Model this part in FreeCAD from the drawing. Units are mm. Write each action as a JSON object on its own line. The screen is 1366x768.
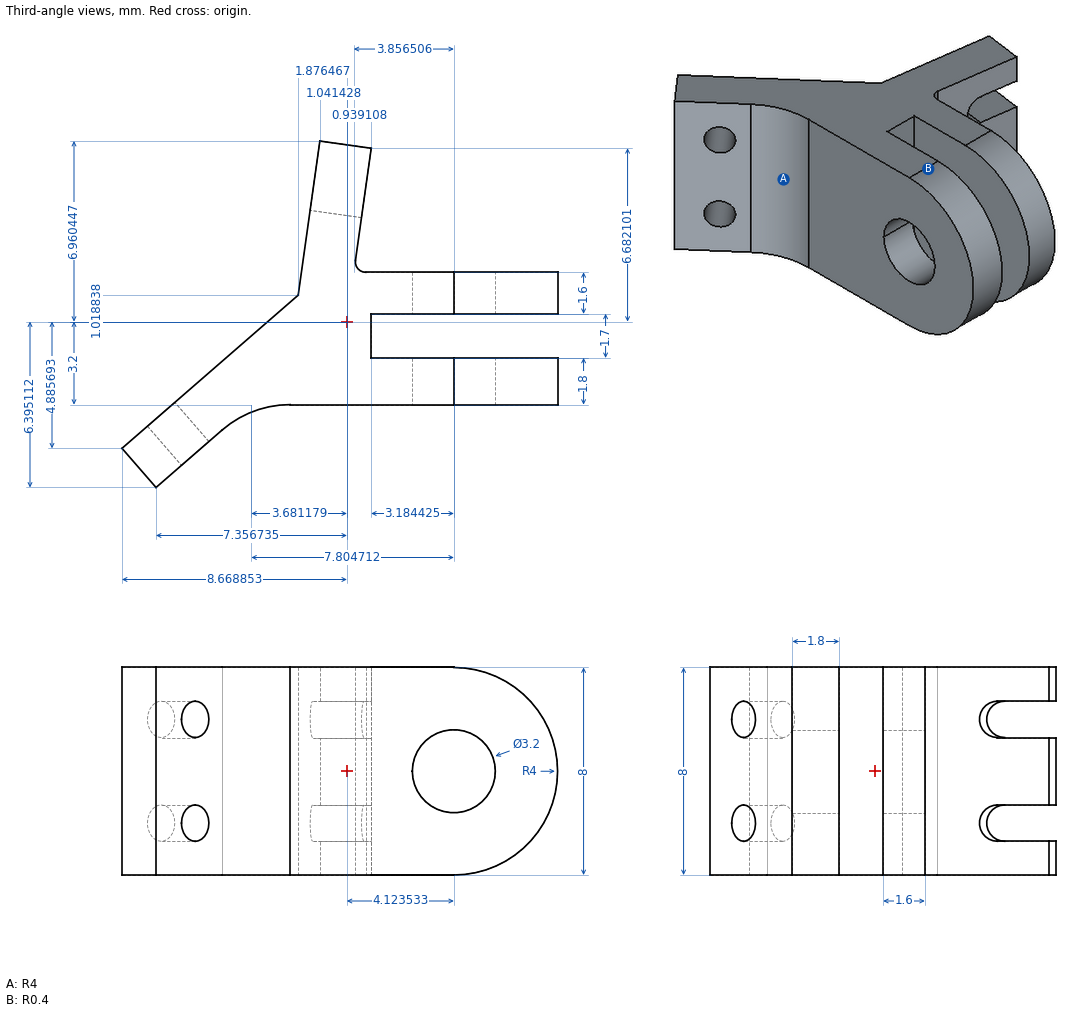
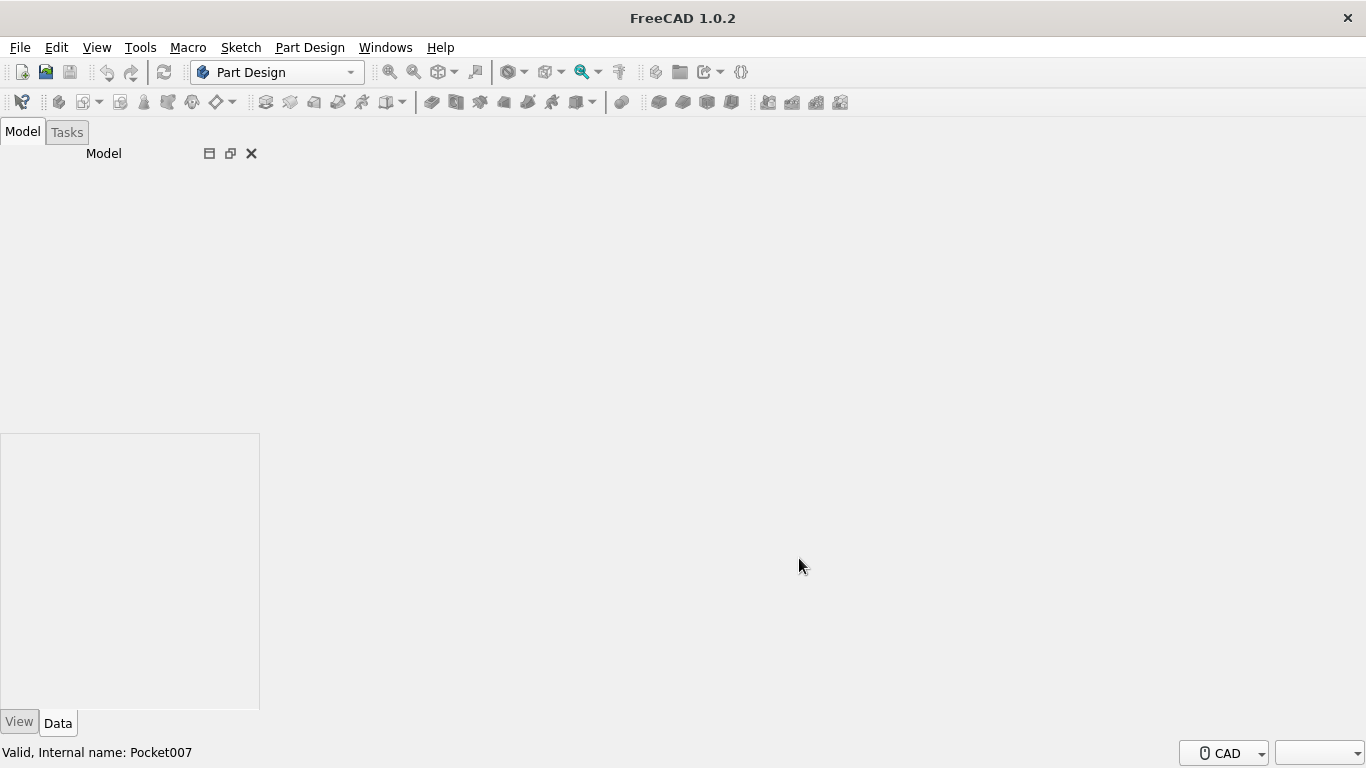
{"action": "left_click", "coordinate": [22, 72]}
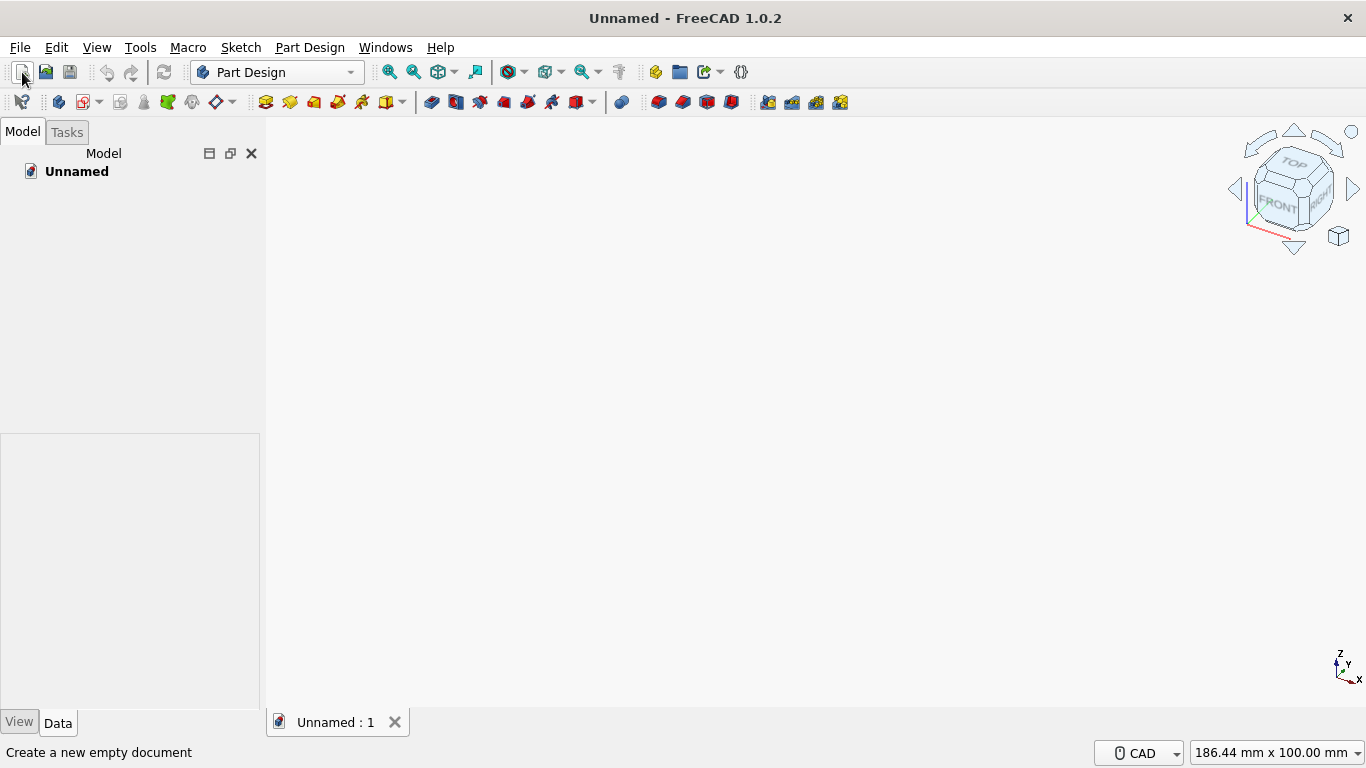
{"action": "left_click", "coordinate": [84, 102]}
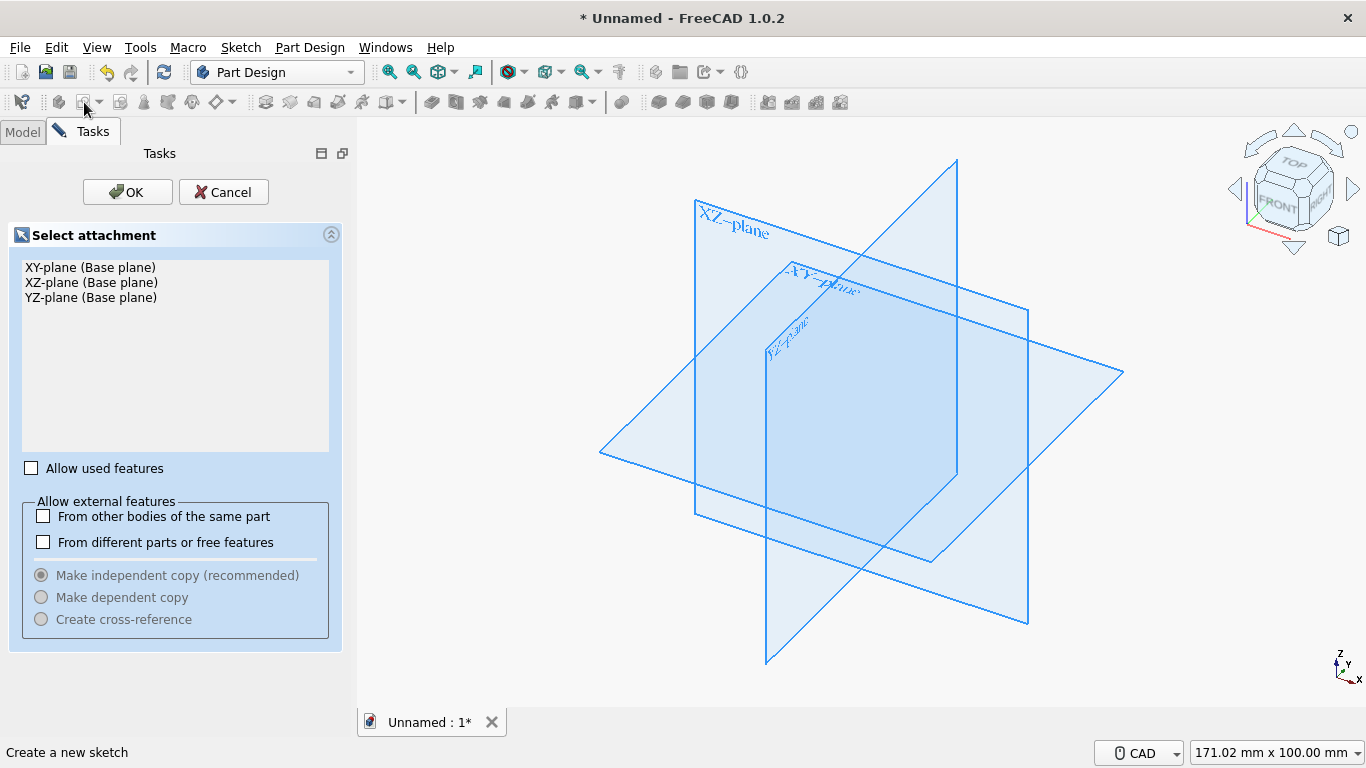
{"action": "left_click", "coordinate": [82, 268]}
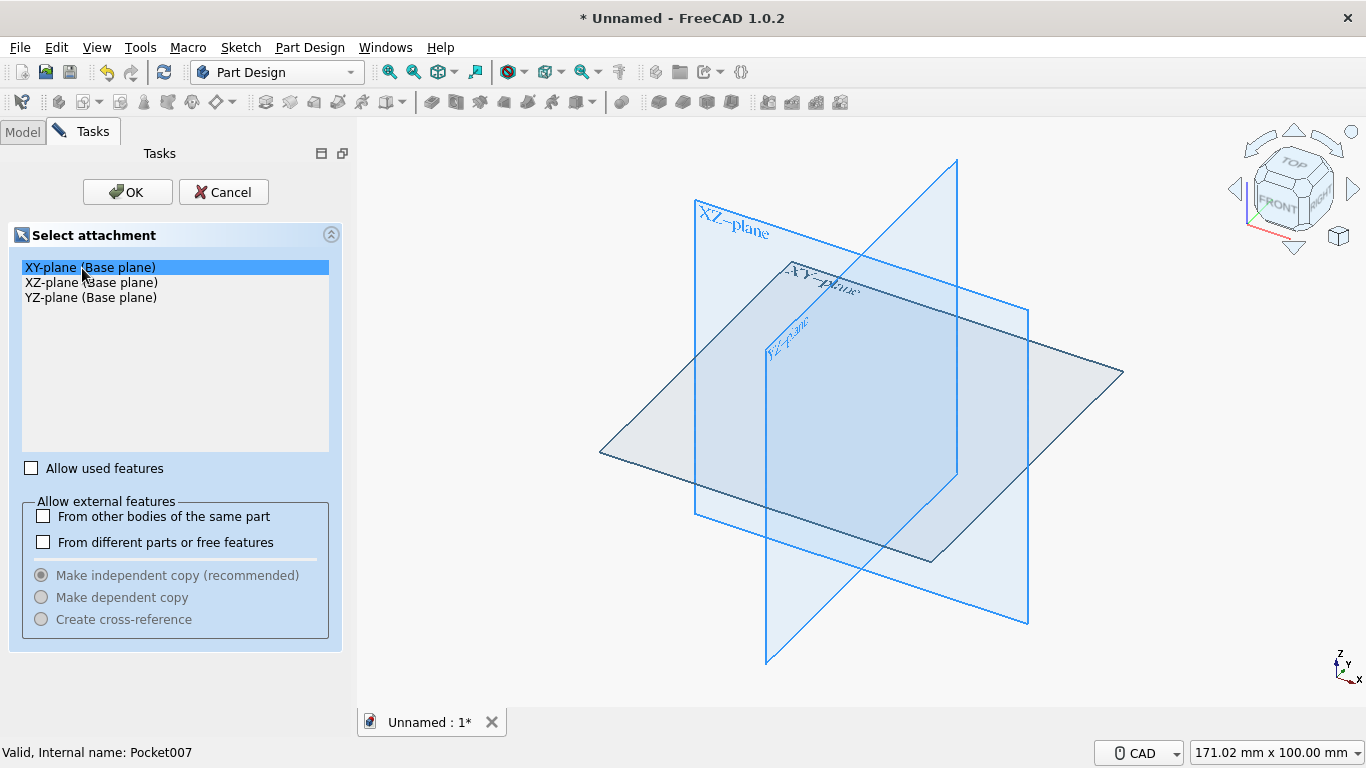
{"action": "left_click", "coordinate": [128, 192]}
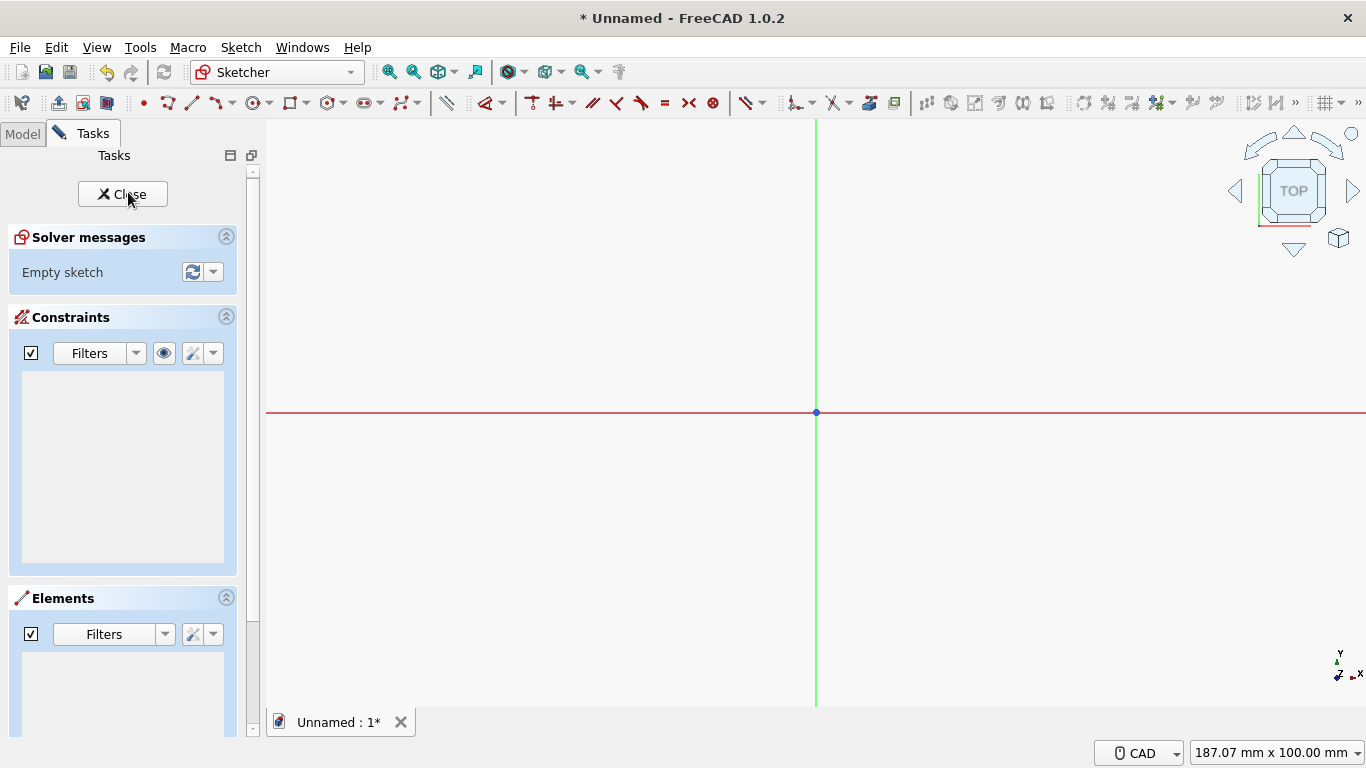
{"action": "scroll", "coordinate": [805, 411], "scroll_direction": "up", "scroll_amount": 8}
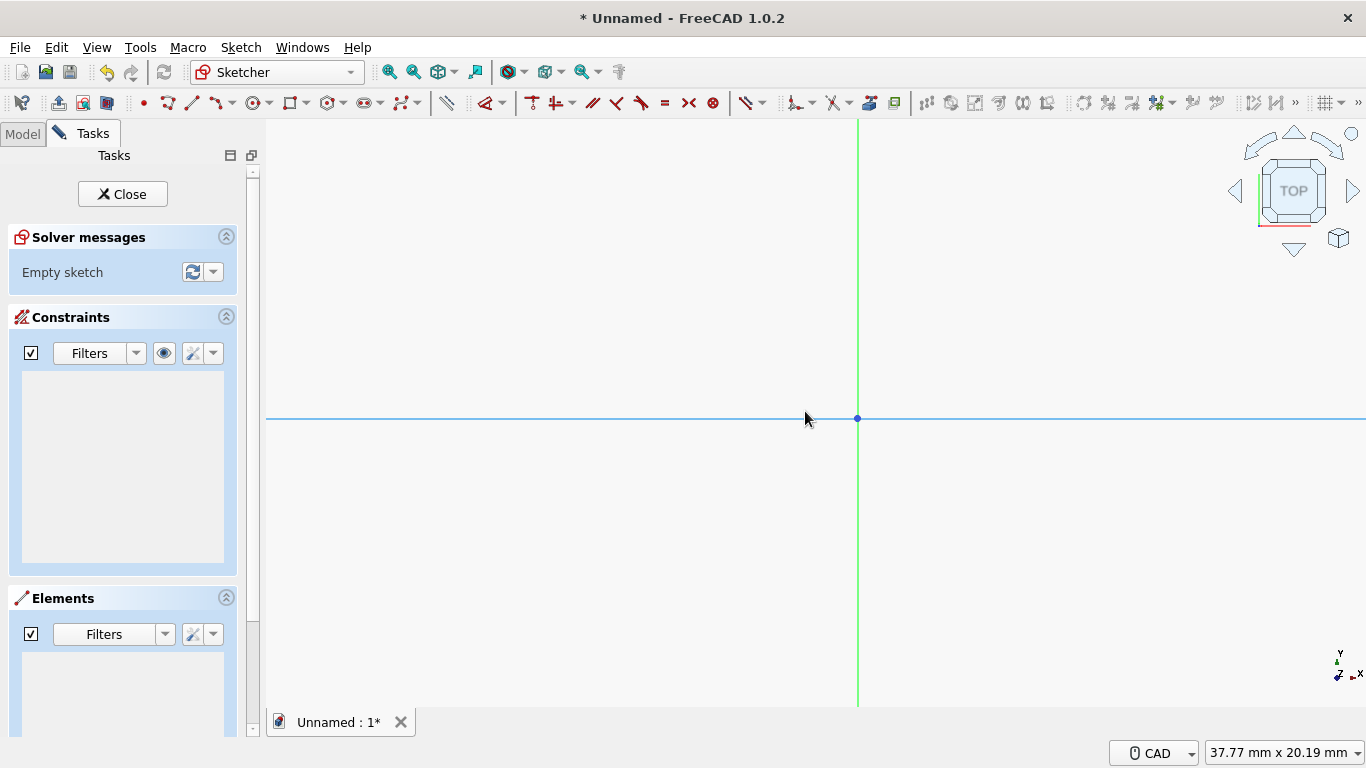
{"action": "left_click", "coordinate": [168, 104]}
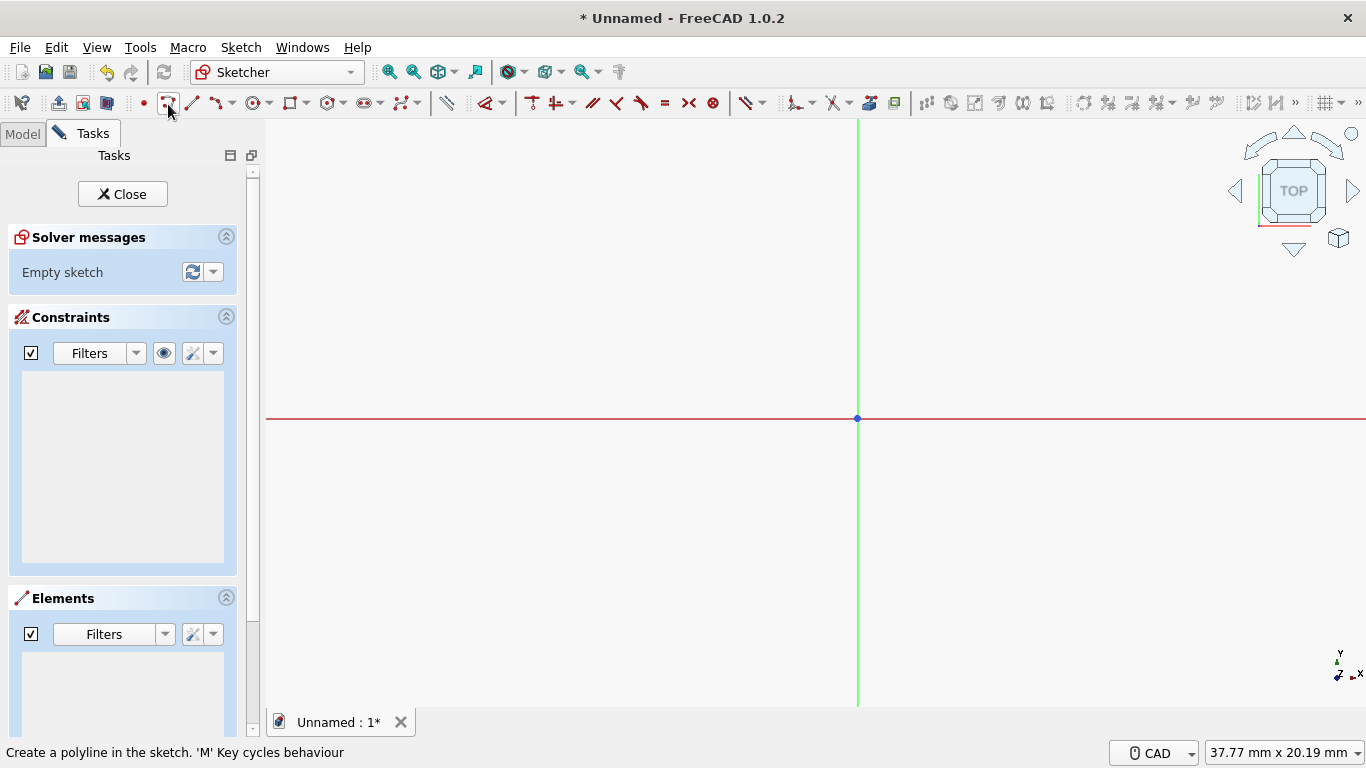
{"action": "left_click", "coordinate": [858, 419]}
{"action": "left_click", "coordinate": [885, 224]}
{"action": "left_click", "coordinate": [827, 216]}
{"action": "left_click", "coordinate": [803, 389]}
{"action": "left_click", "coordinate": [605, 561]}
{"action": "left_click", "coordinate": [643, 605]}
{"action": "left_click", "coordinate": [858, 419]}
{"action": "key", "text": "Escape"}
{"action": "key", "text": "Escape"}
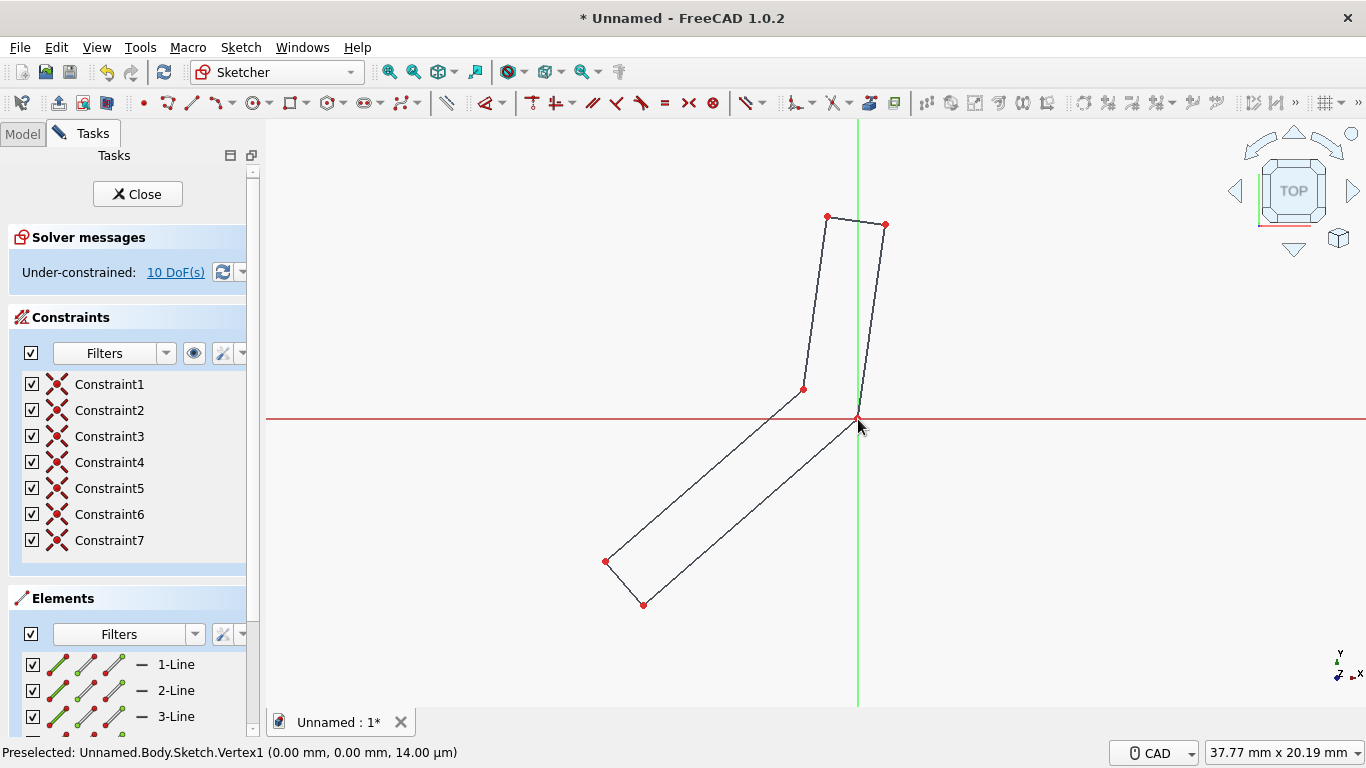
{"action": "left_click", "coordinate": [486, 104]}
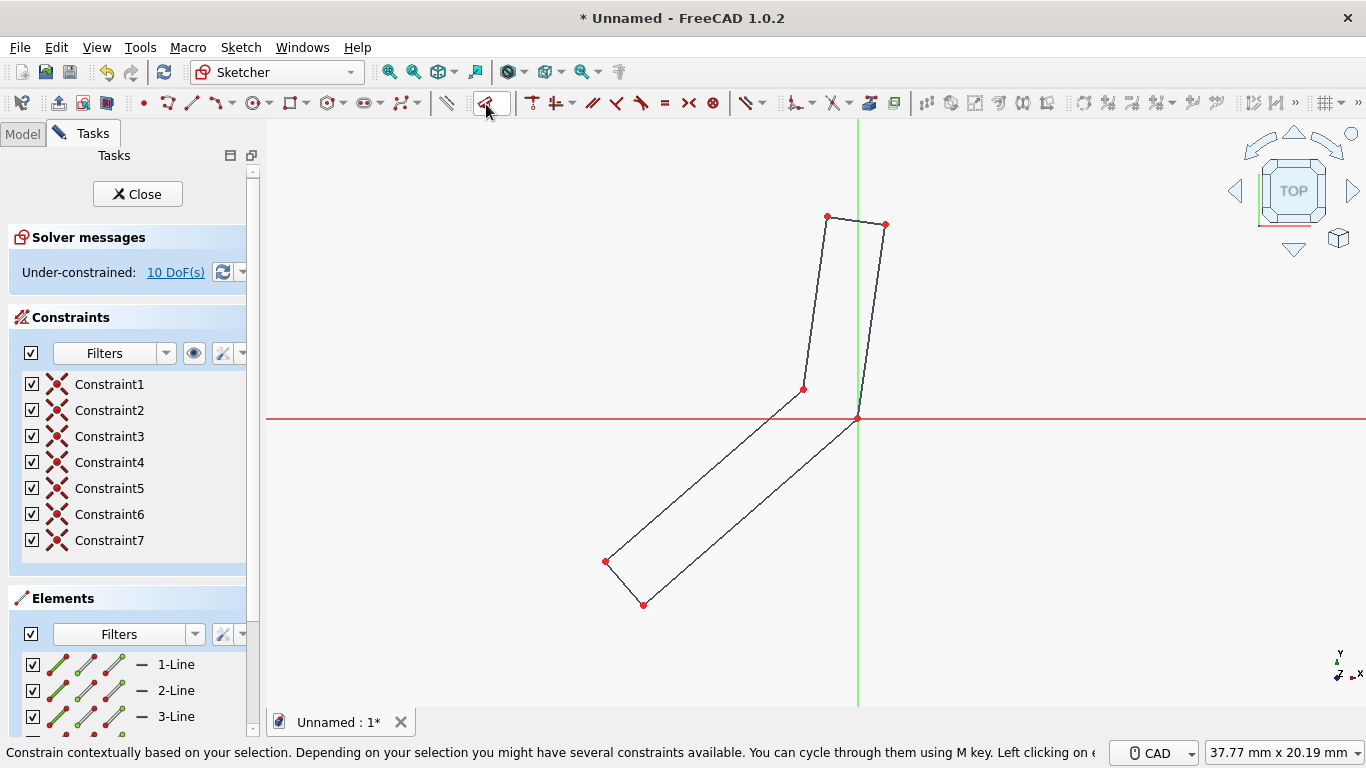
{"action": "scroll", "coordinate": [885, 225], "scroll_direction": "up", "scroll_amount": 2}